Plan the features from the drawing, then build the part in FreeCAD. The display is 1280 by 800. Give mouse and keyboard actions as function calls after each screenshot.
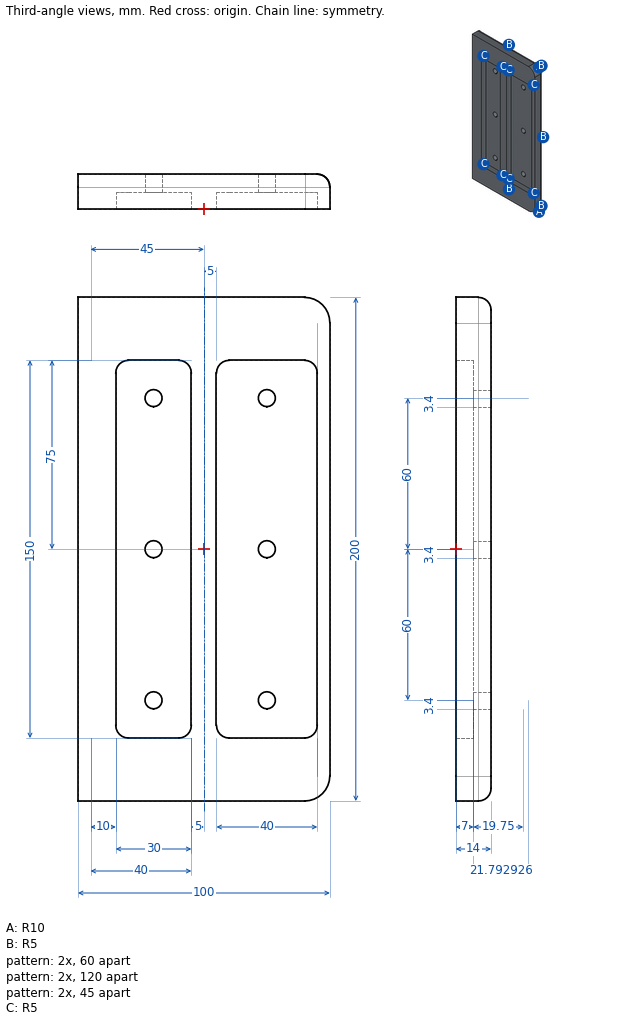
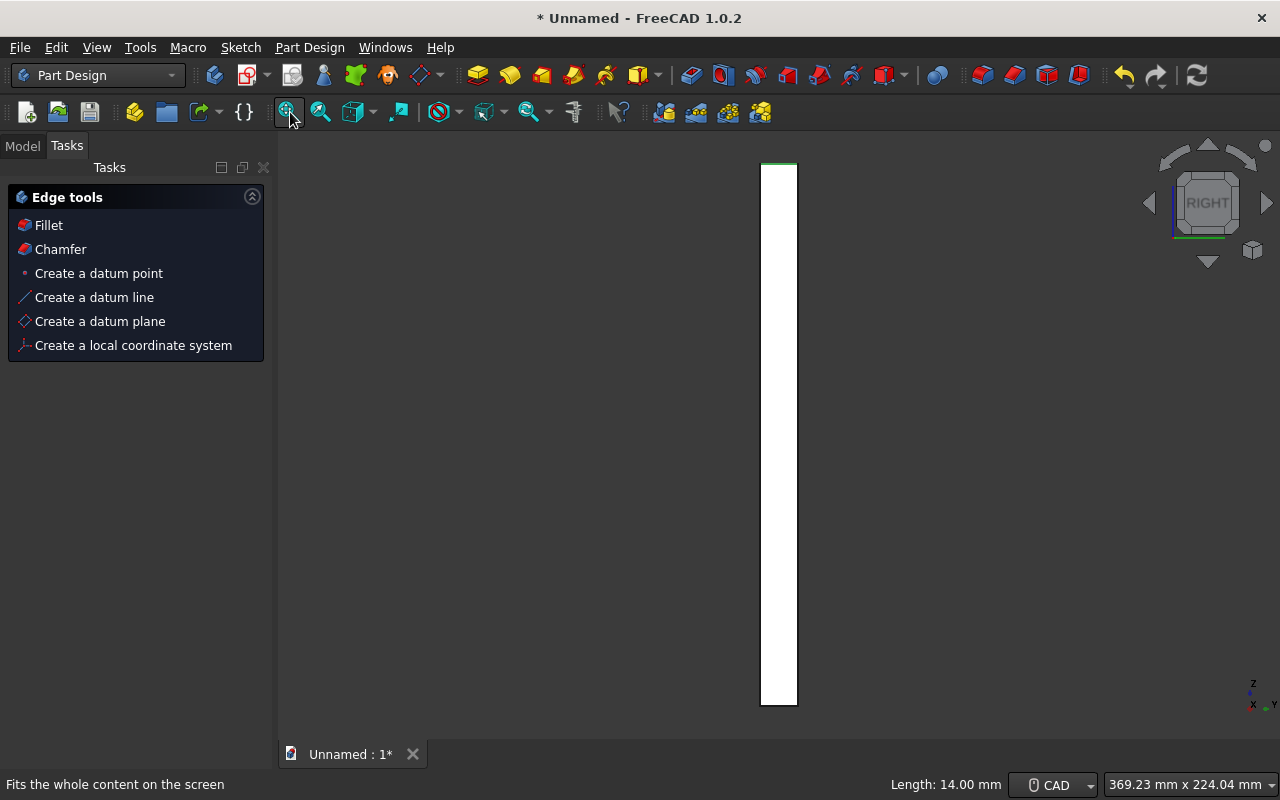
click(779, 705, ctrl)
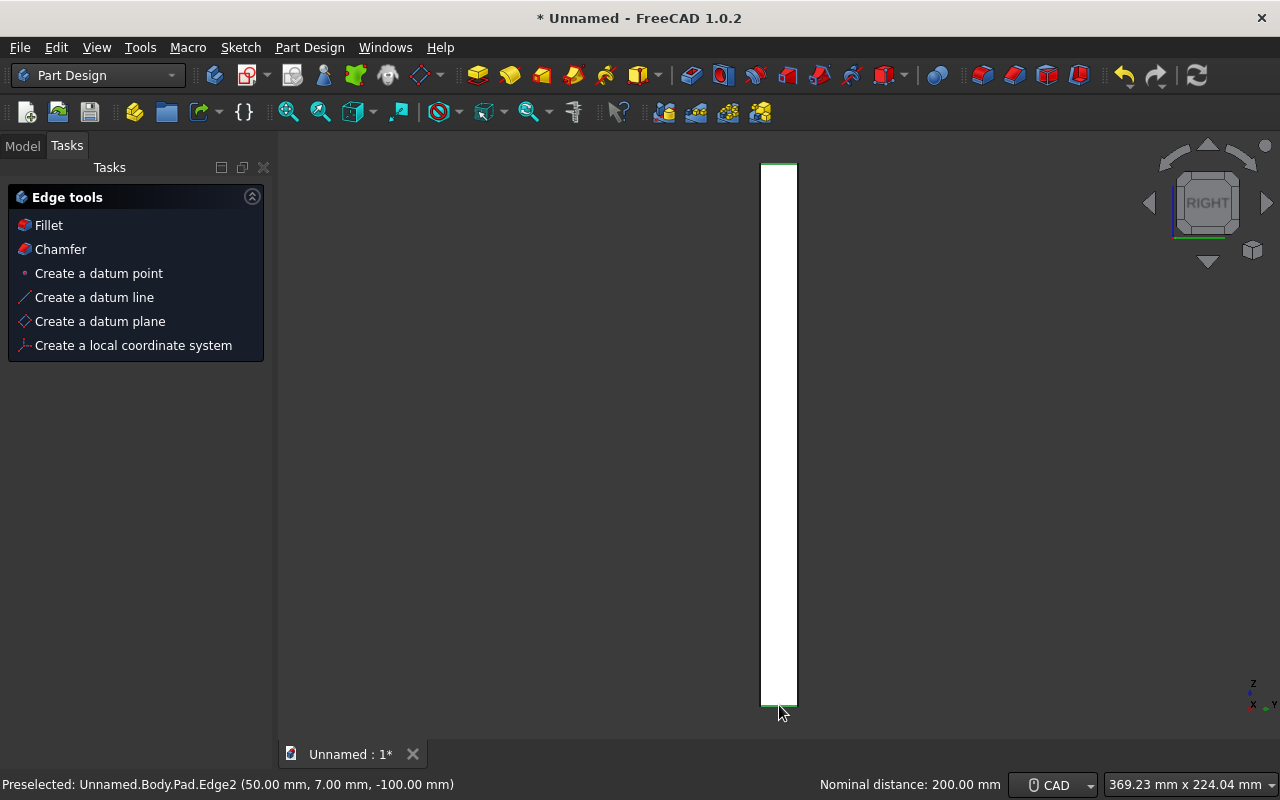
click(984, 76)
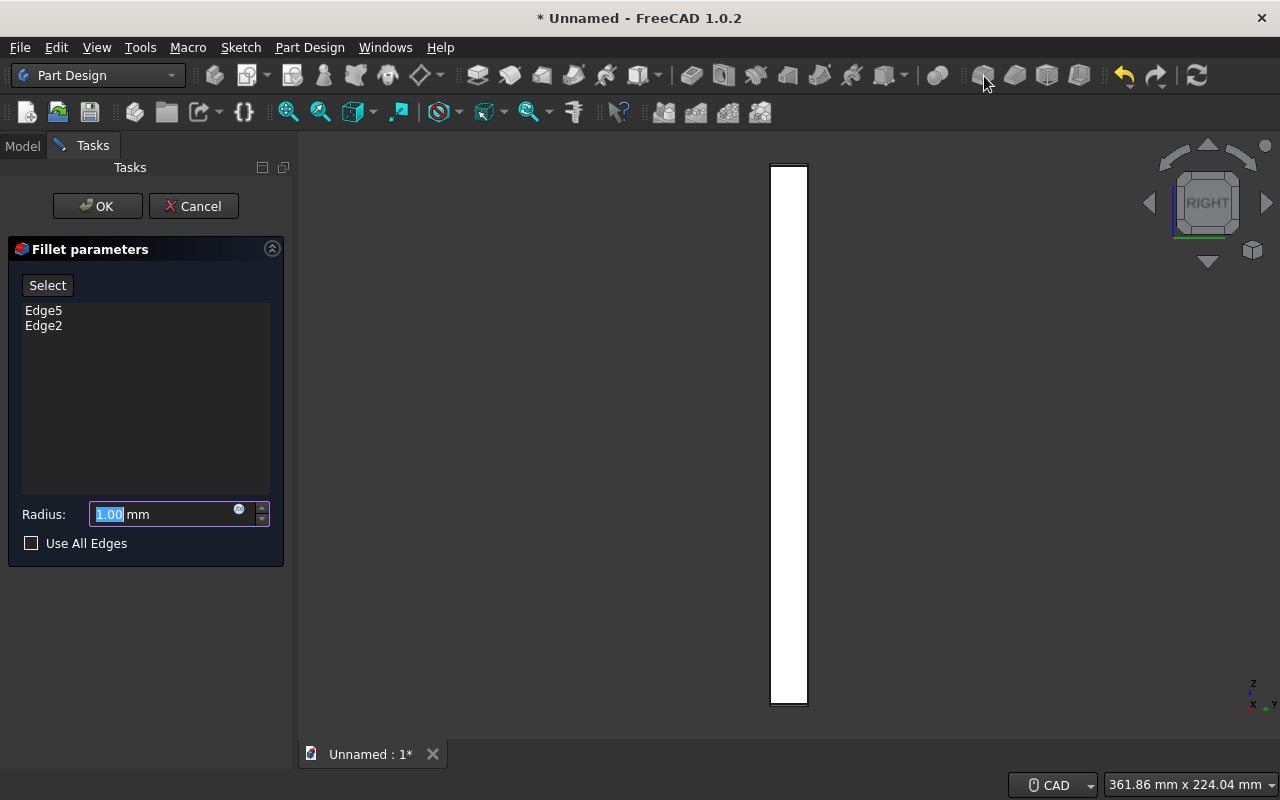
text(10)
key(Tab)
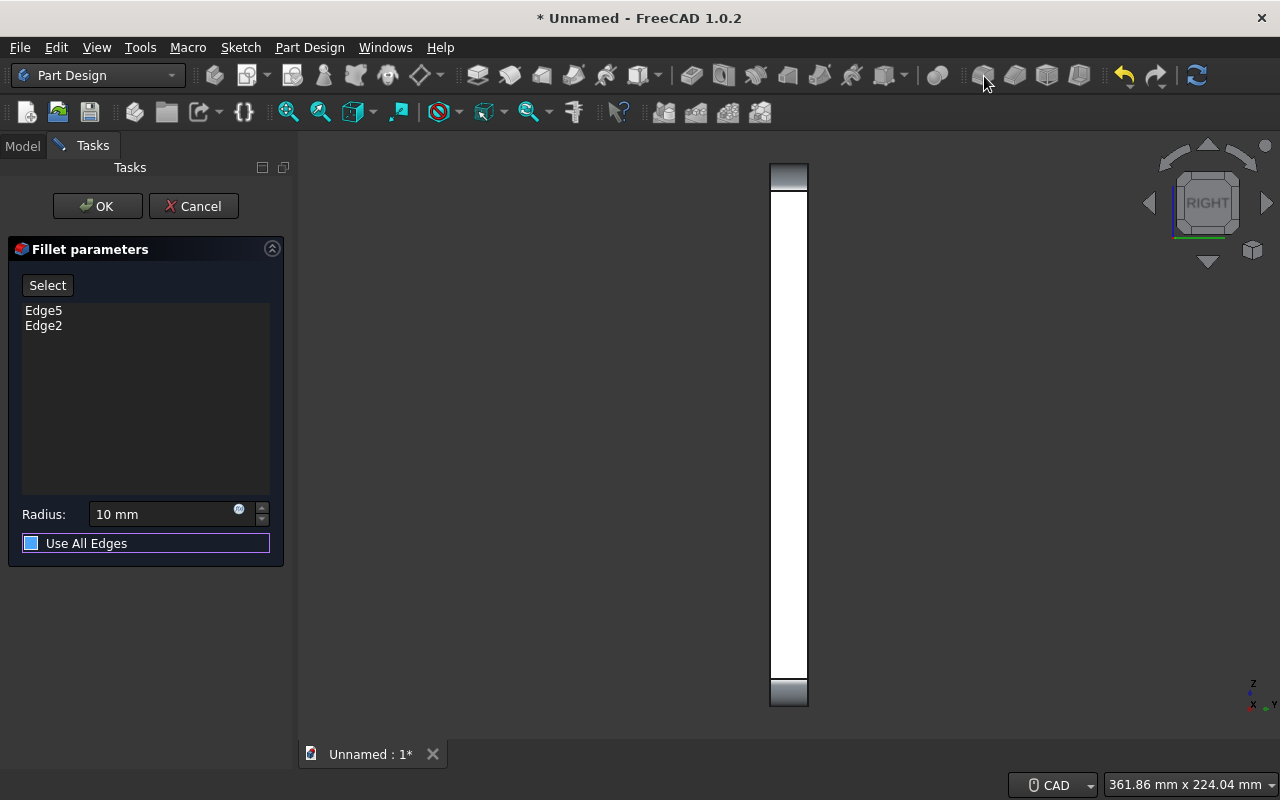
click(98, 206)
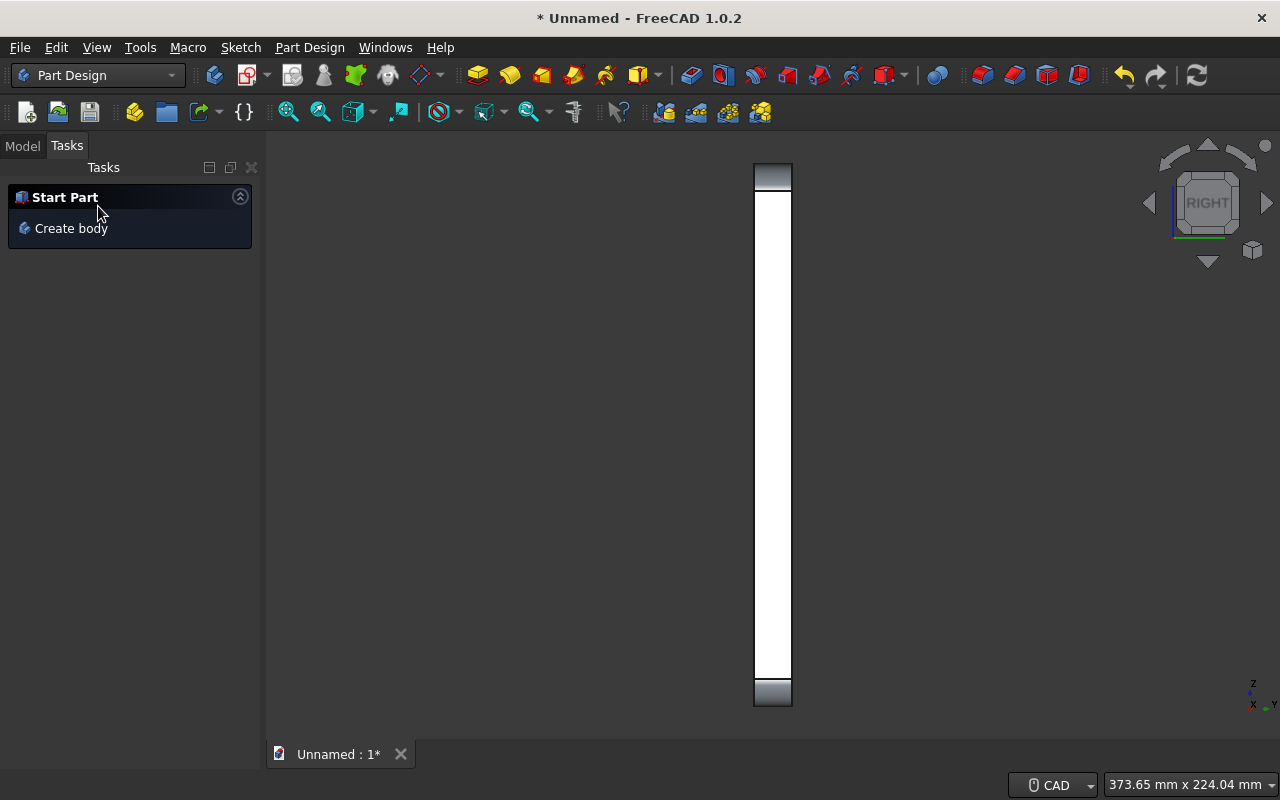
click(792, 434)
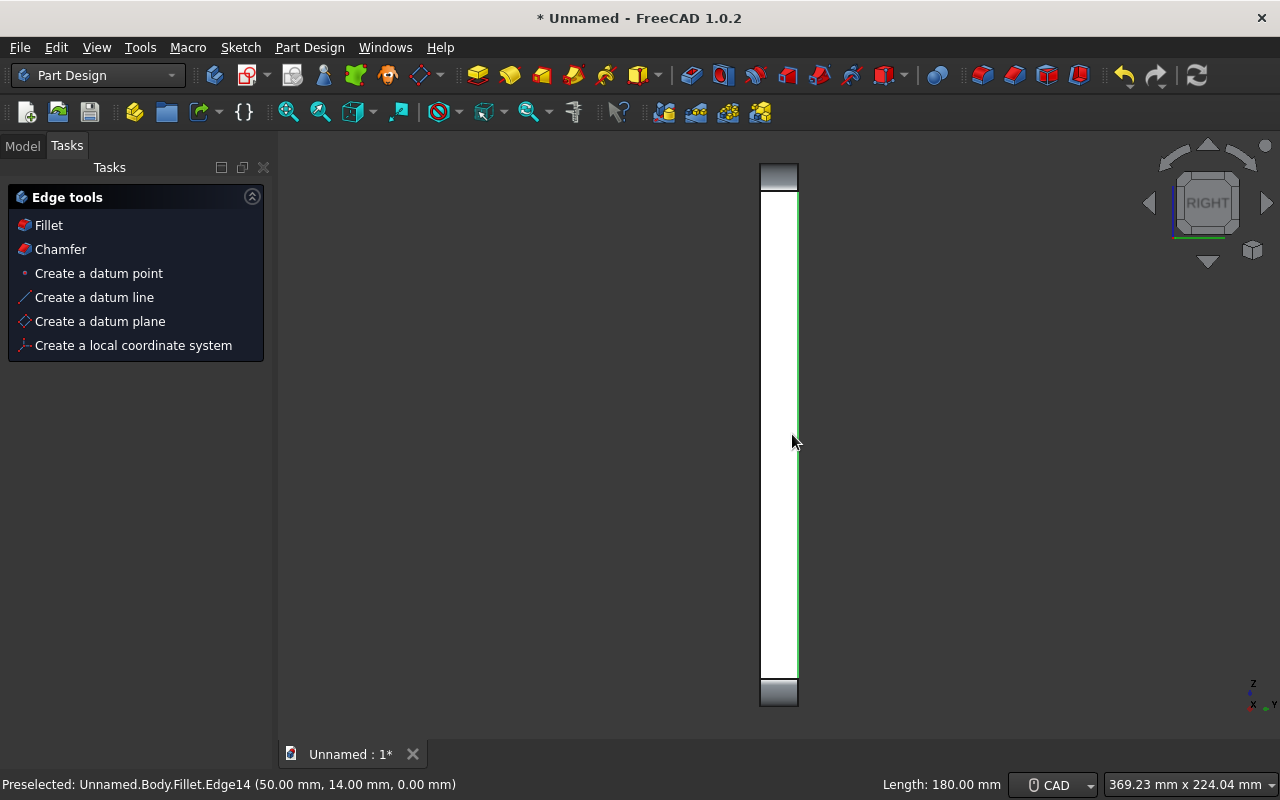
click(798, 171, ctrl)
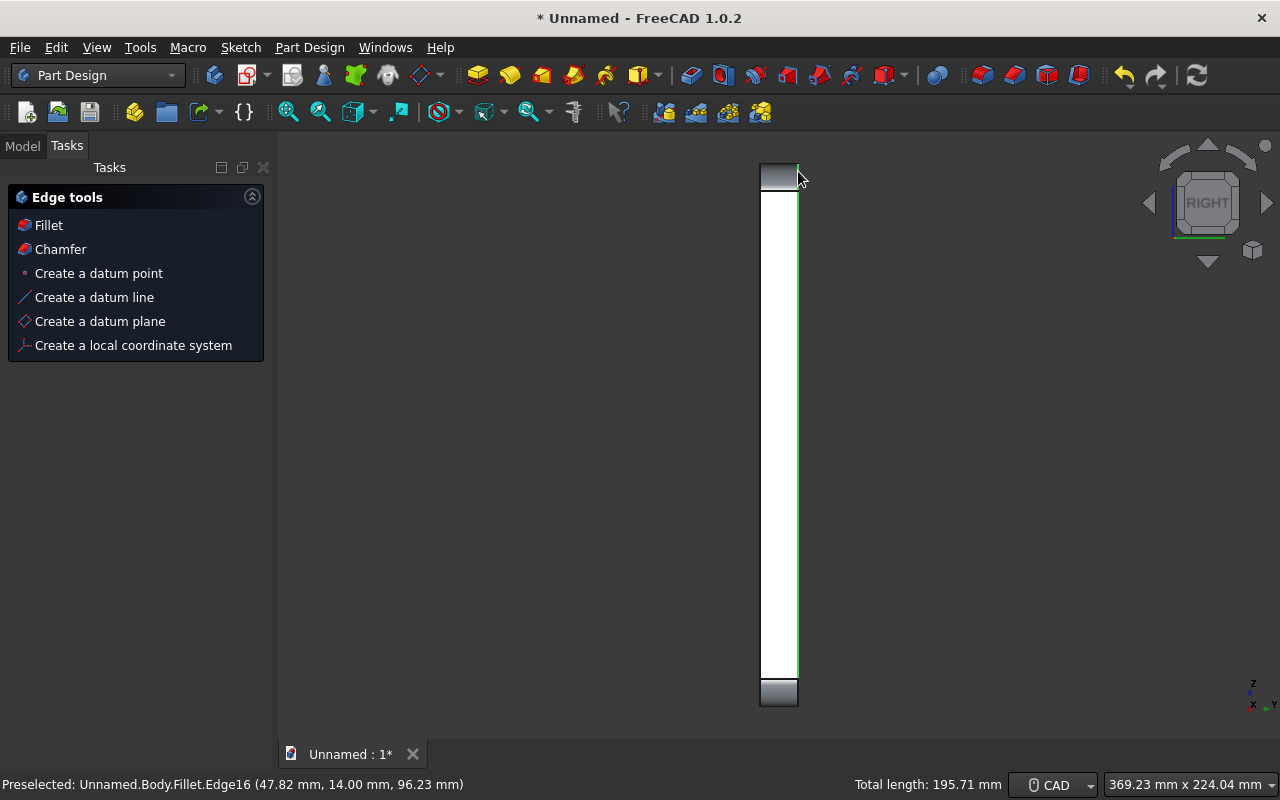
click(798, 697, ctrl)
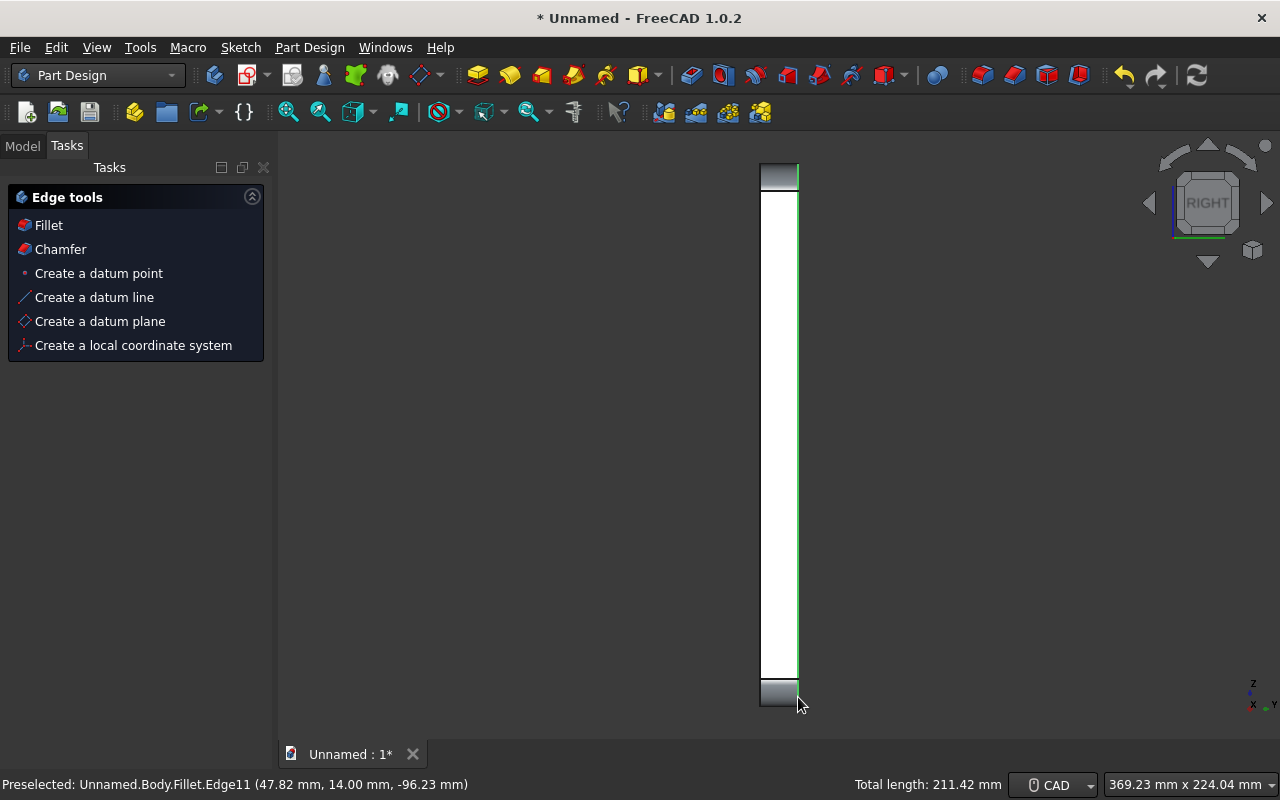
key(0)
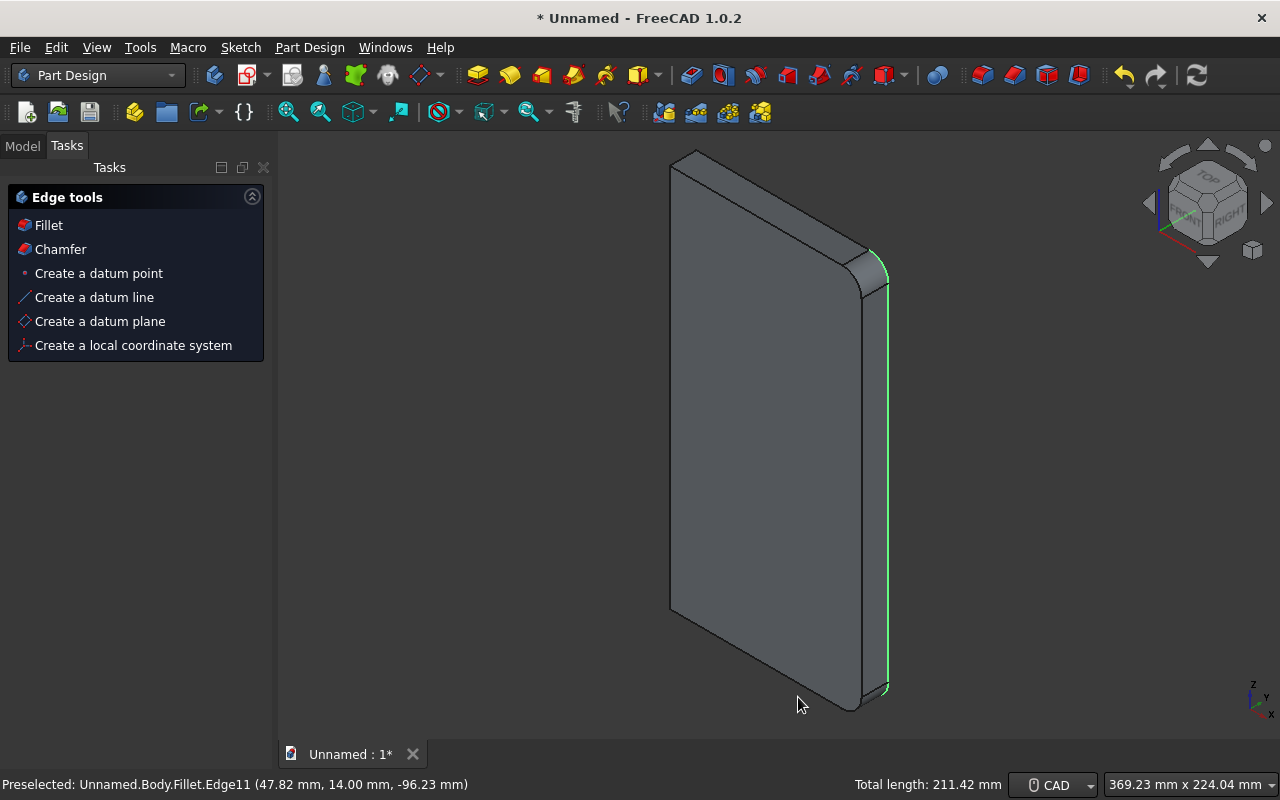
key(2)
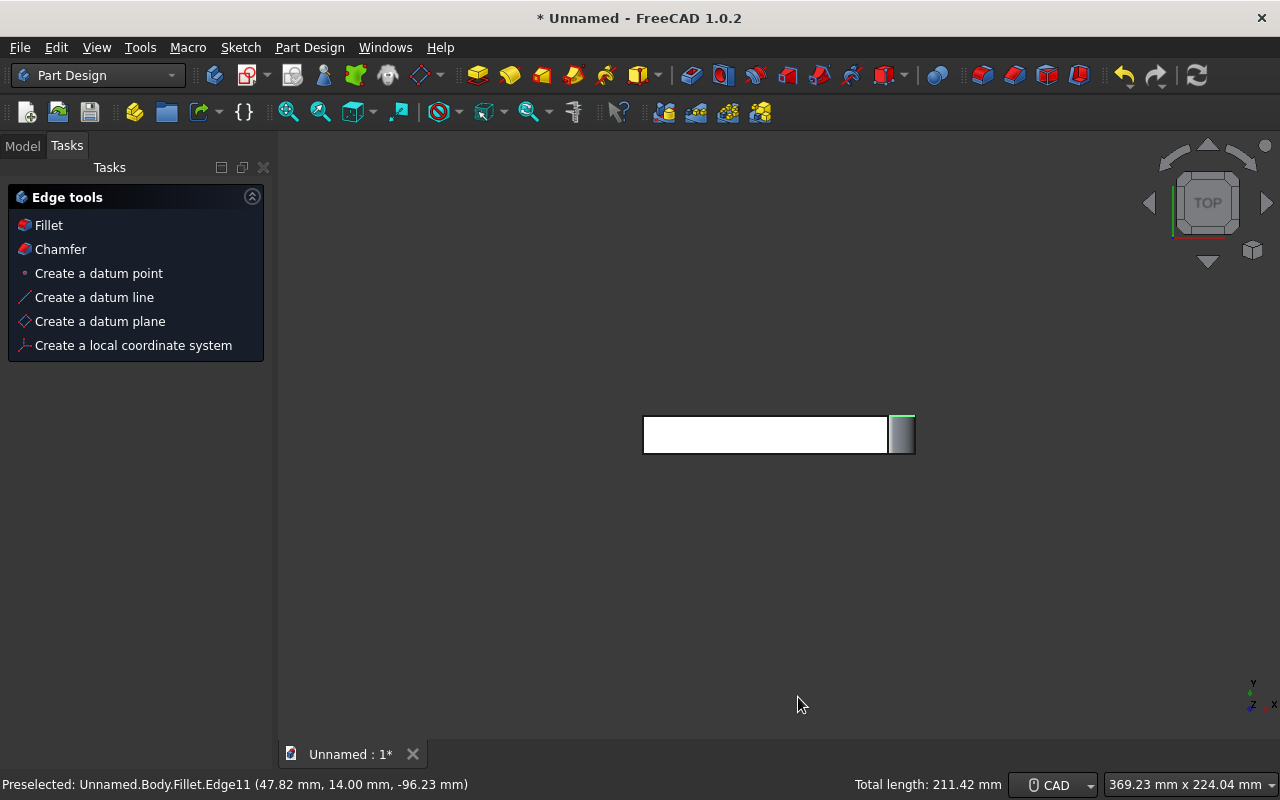
key(v)
key(f)